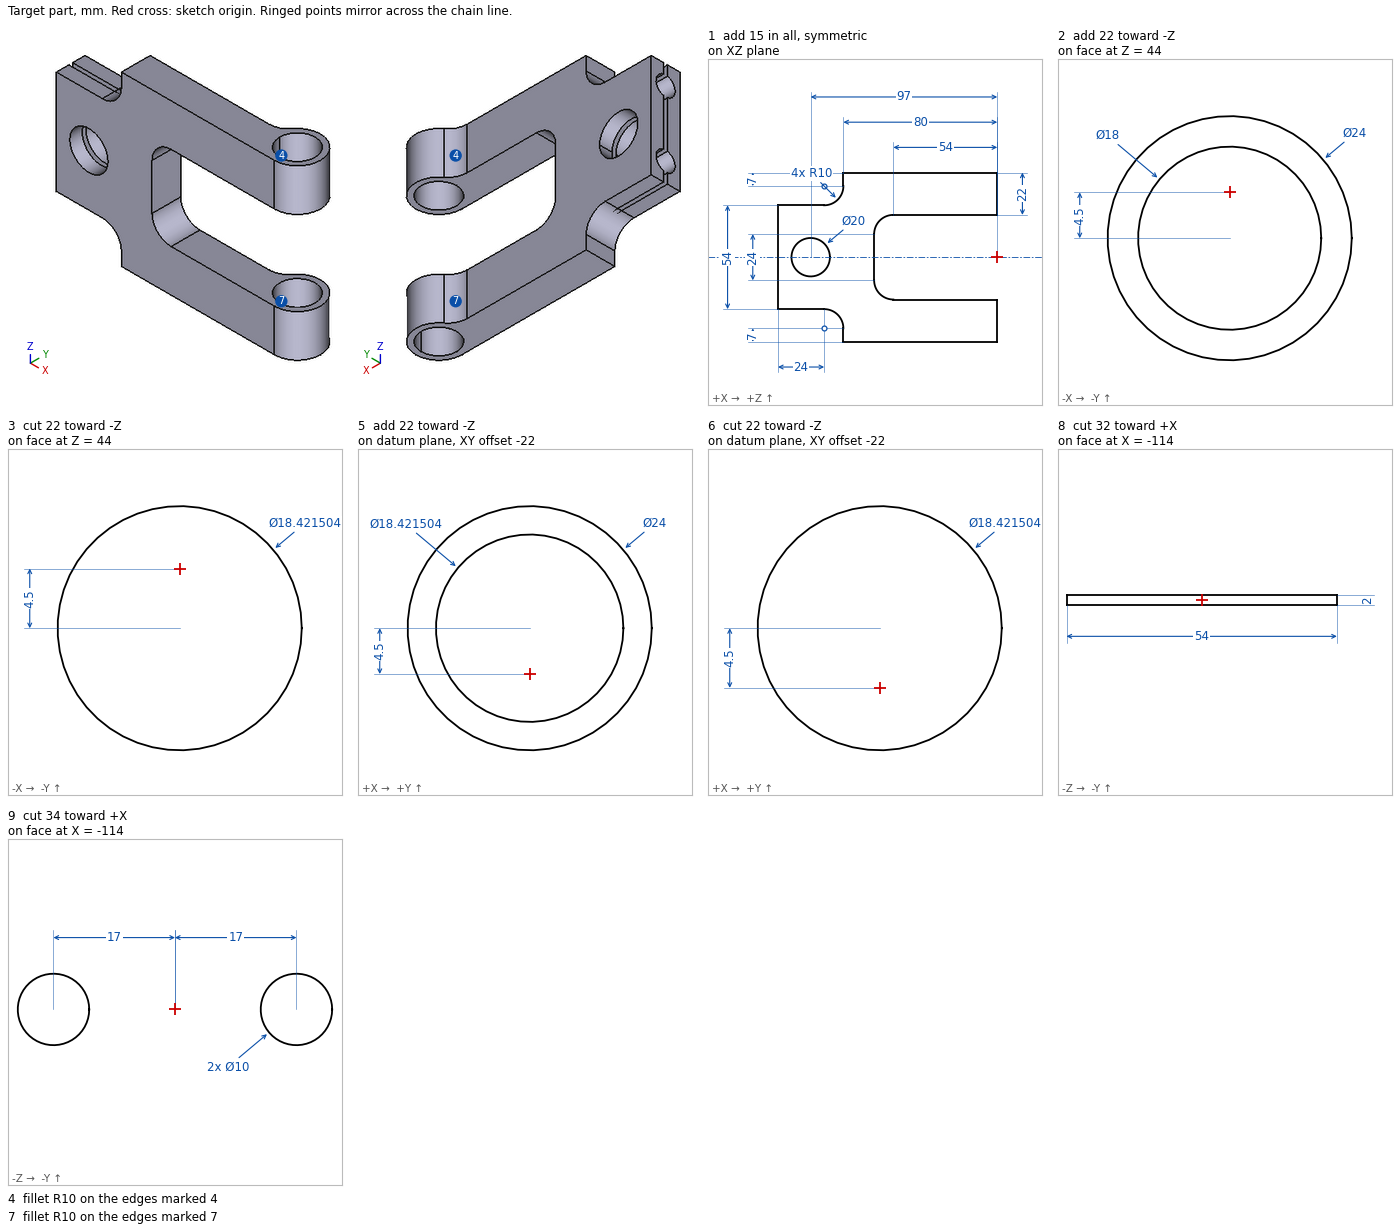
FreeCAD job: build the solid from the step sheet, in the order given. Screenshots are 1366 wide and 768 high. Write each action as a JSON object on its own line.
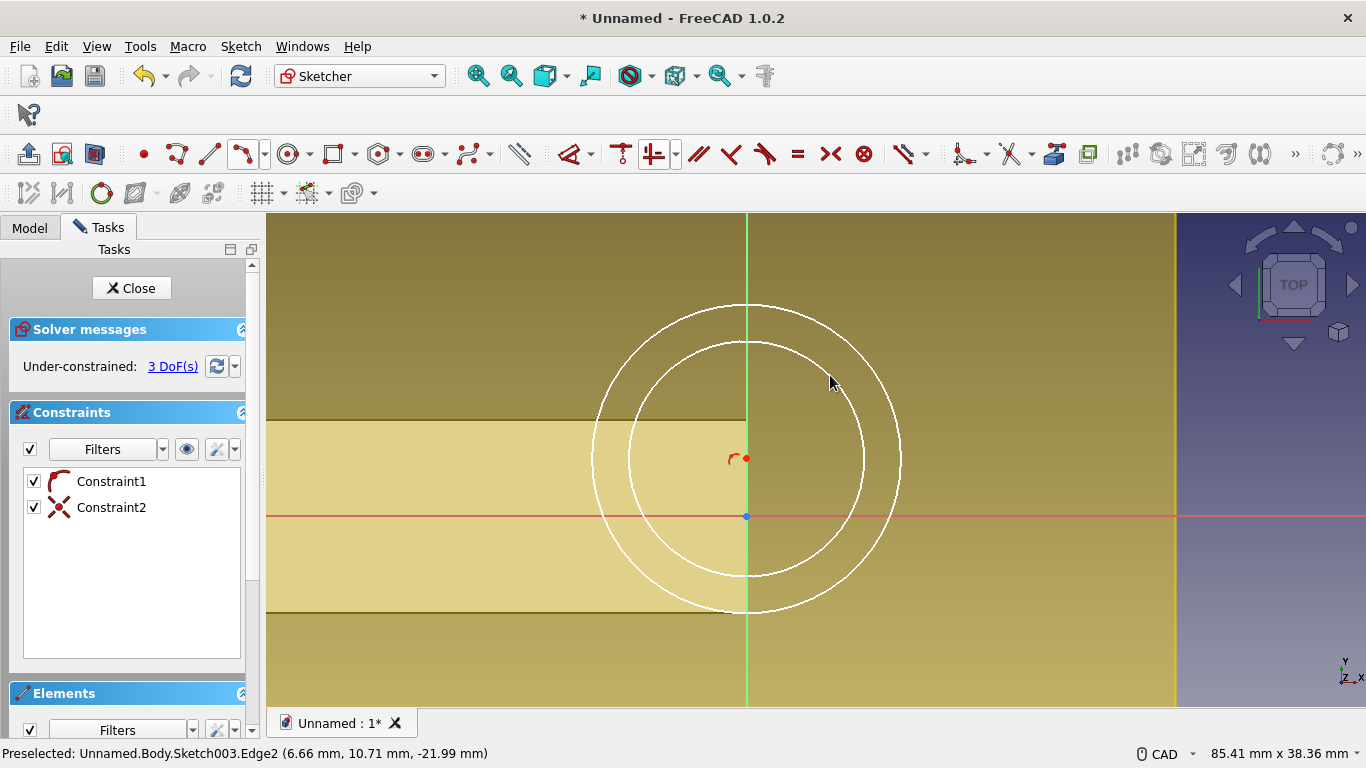
{"action": "left_click", "coordinate": [568, 154]}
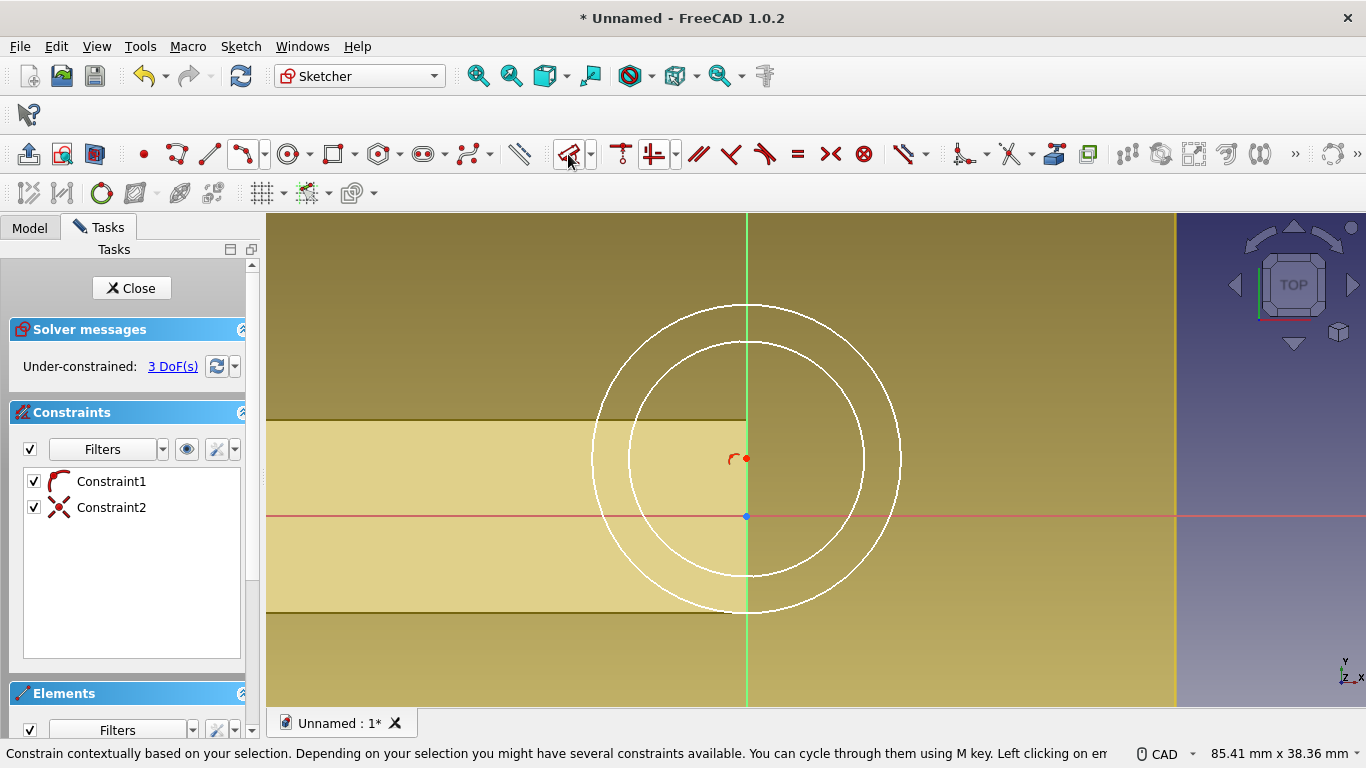
{"action": "left_click", "coordinate": [855, 349]}
{"action": "left_click", "coordinate": [877, 326]}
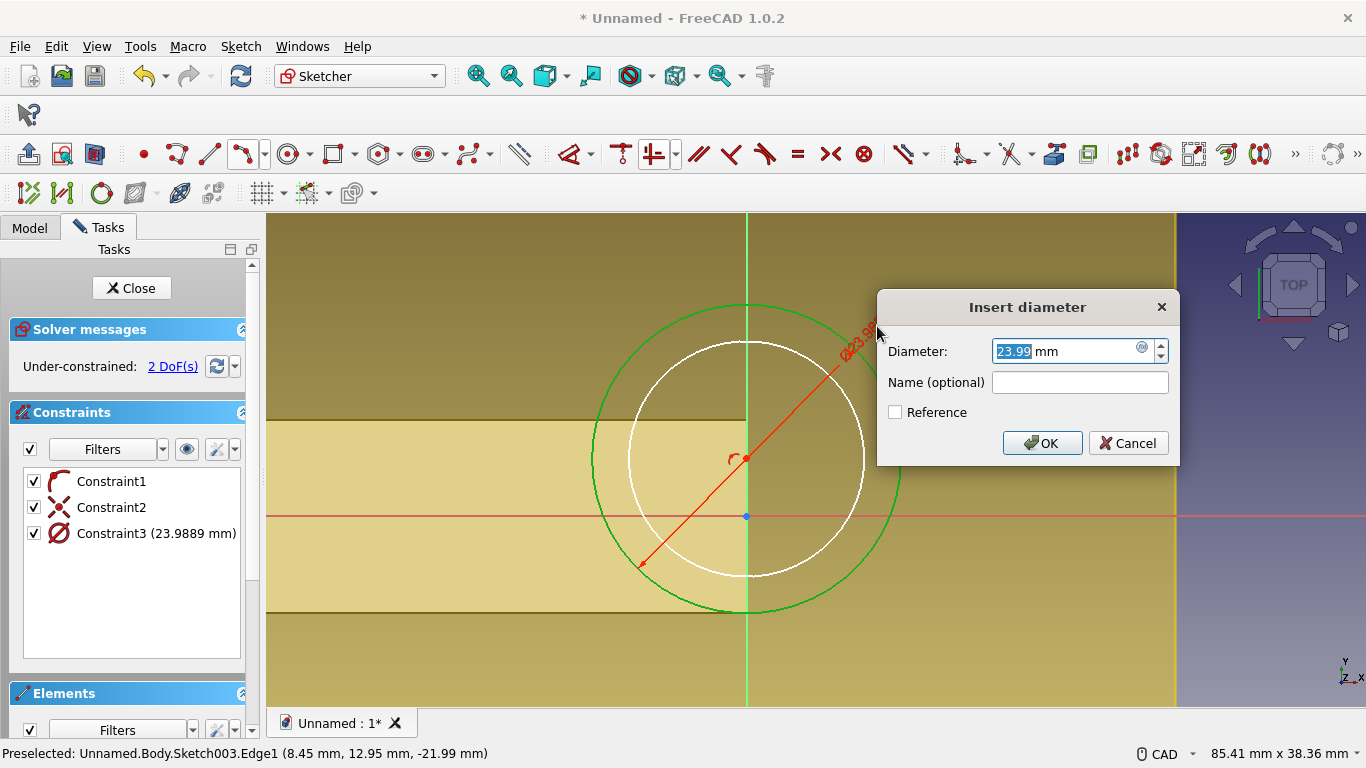
{"action": "type", "text": "24"}
{"action": "key", "text": "Return"}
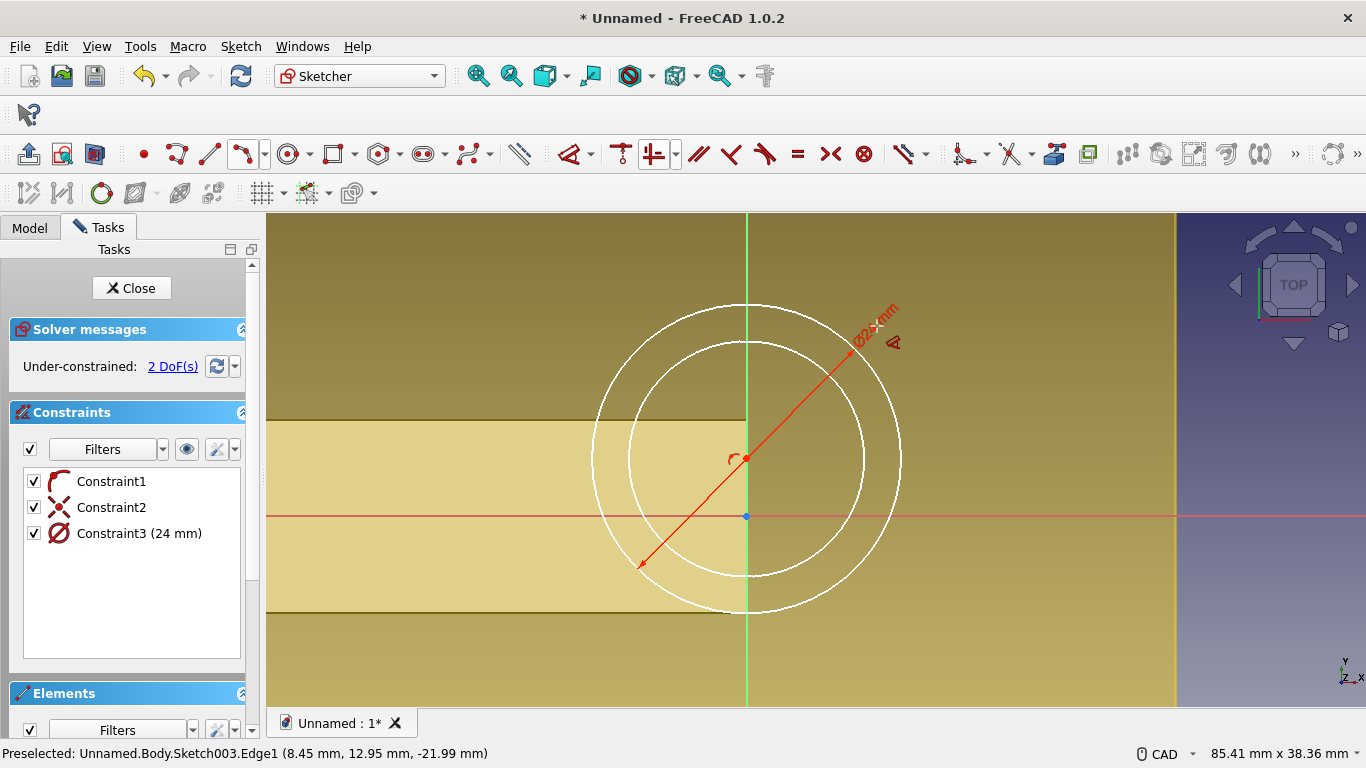
{"action": "left_click", "coordinate": [830, 376]}
{"action": "left_click", "coordinate": [912, 411]}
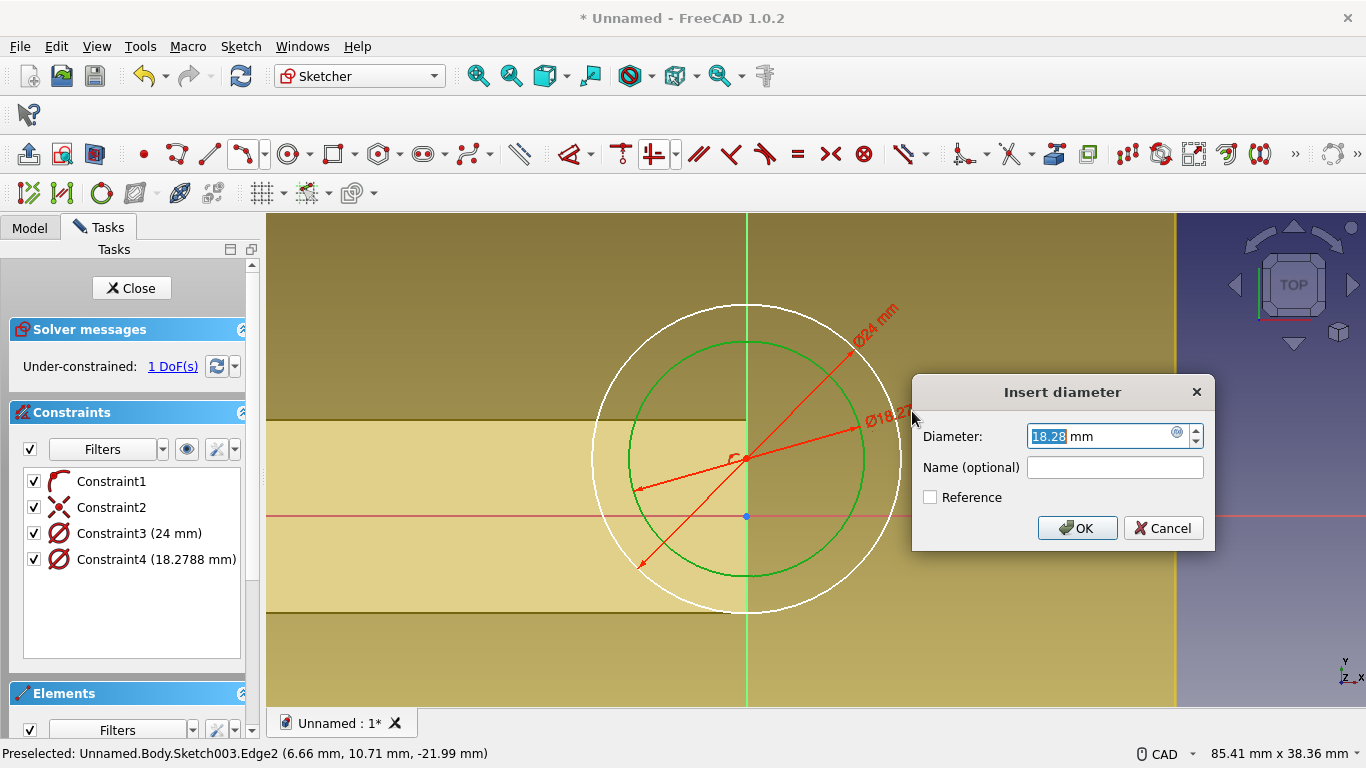
{"action": "type", "text": "18.421504"}
{"action": "key", "text": "Return"}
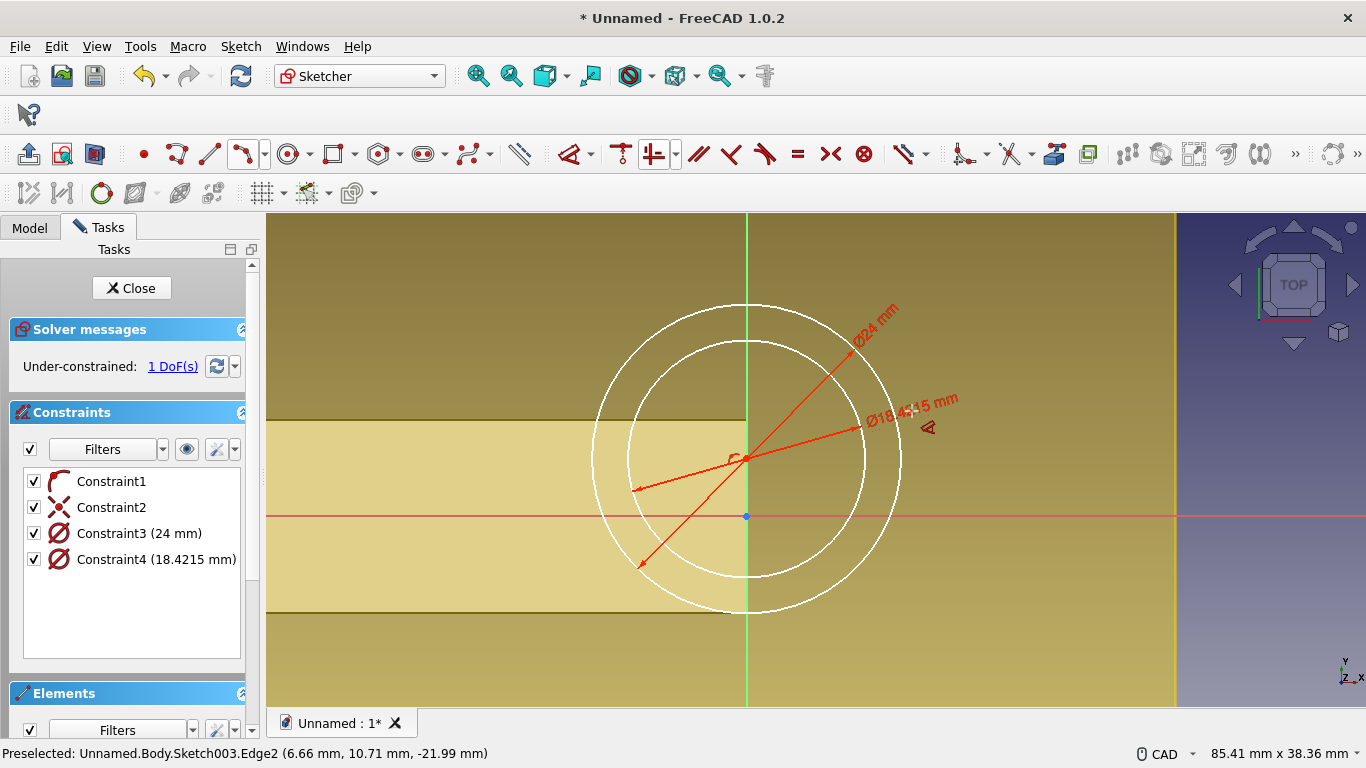
{"action": "left_click", "coordinate": [747, 459]}
{"action": "left_click", "coordinate": [781, 488]}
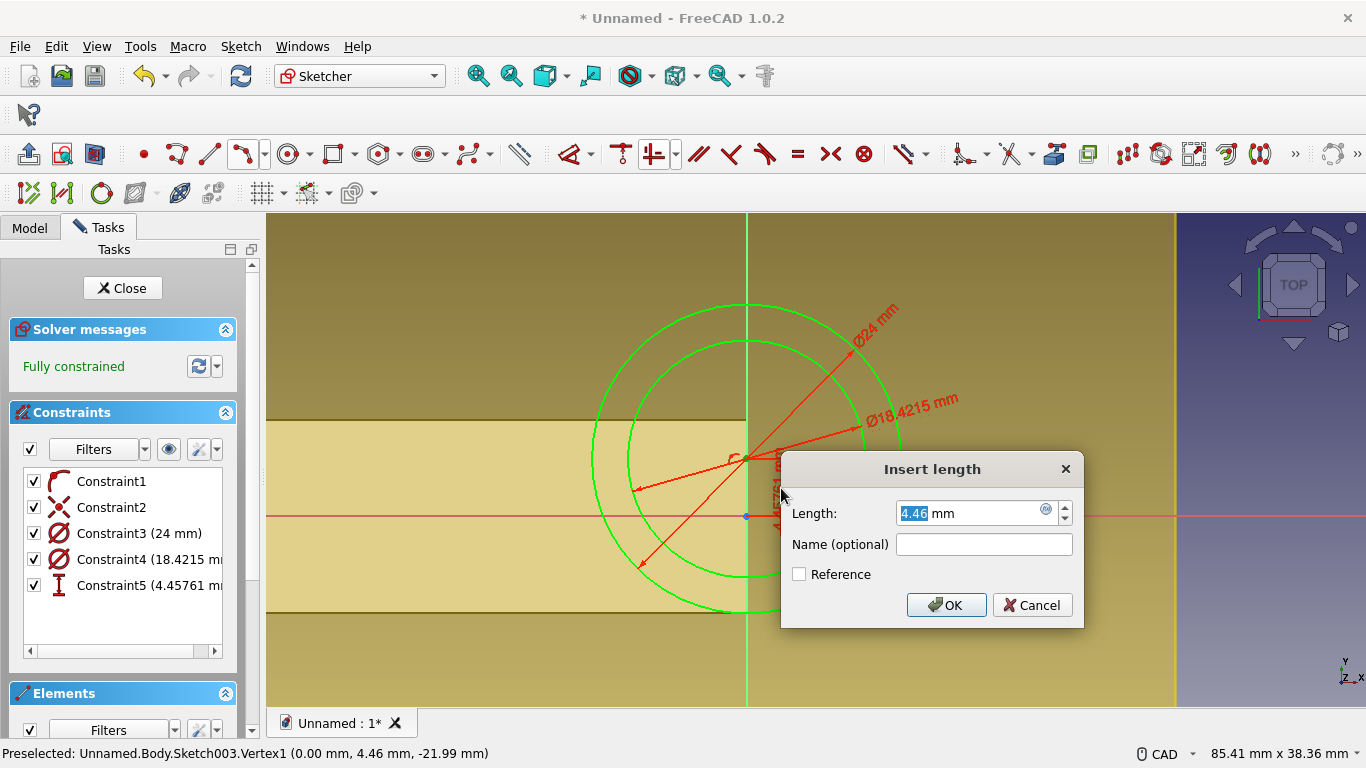
{"action": "type", "text": "4.5"}
{"action": "key", "text": "Return"}
{"action": "key", "text": "Escape"}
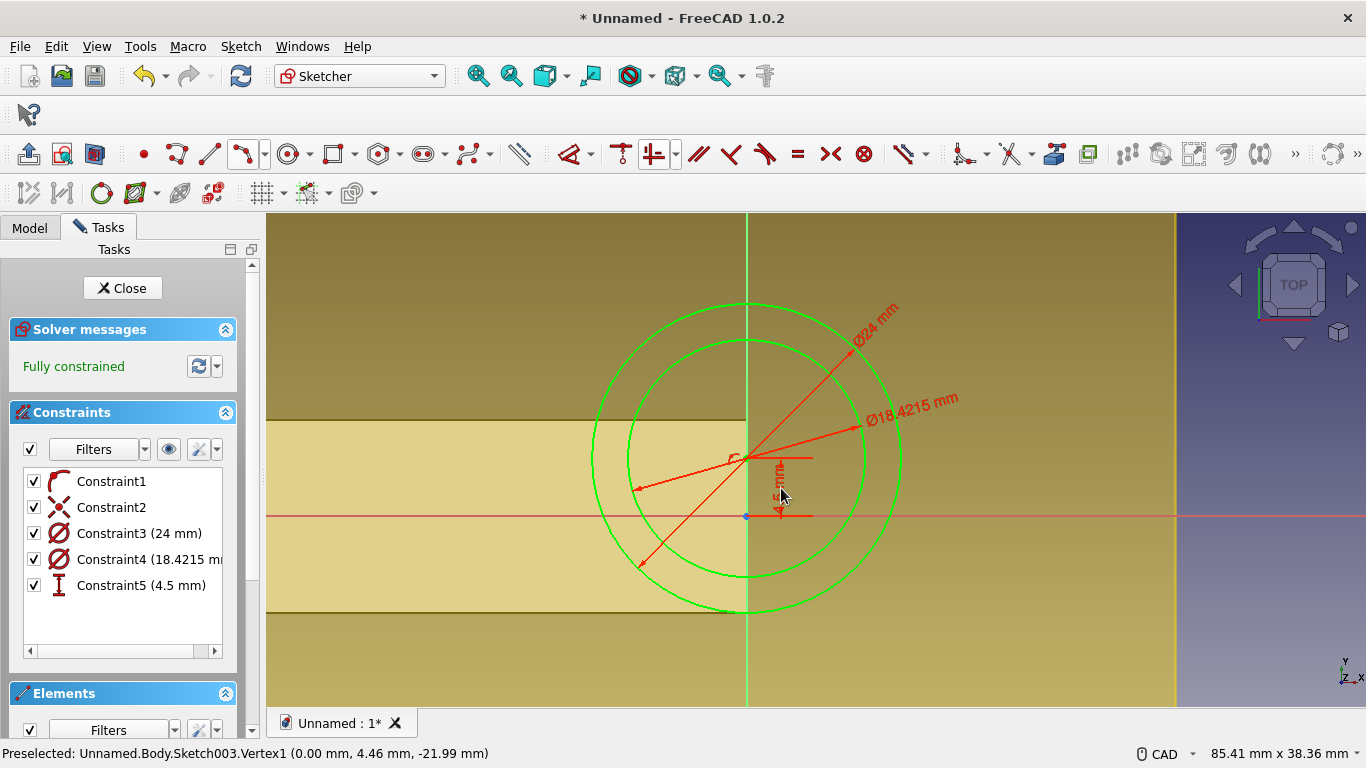
{"action": "left_click", "coordinate": [123, 288]}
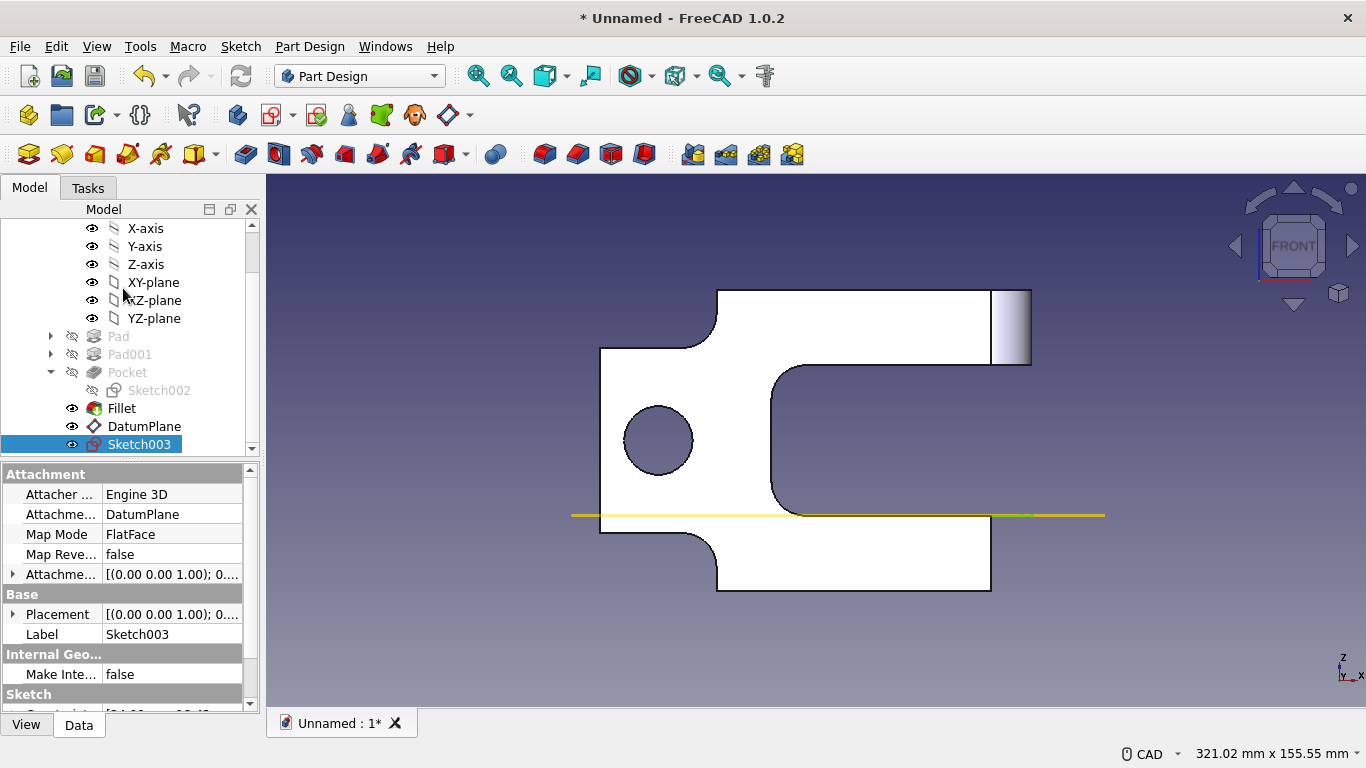
{"action": "left_click", "coordinate": [29, 154]}